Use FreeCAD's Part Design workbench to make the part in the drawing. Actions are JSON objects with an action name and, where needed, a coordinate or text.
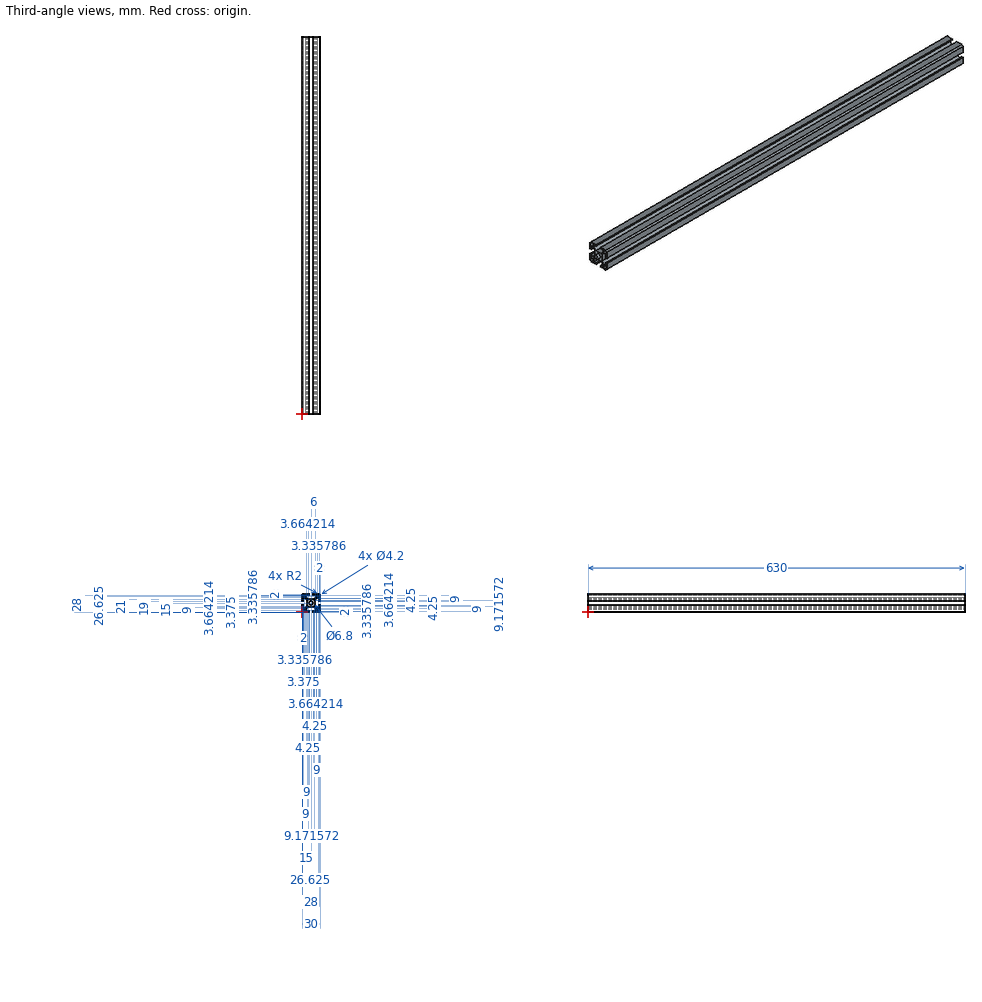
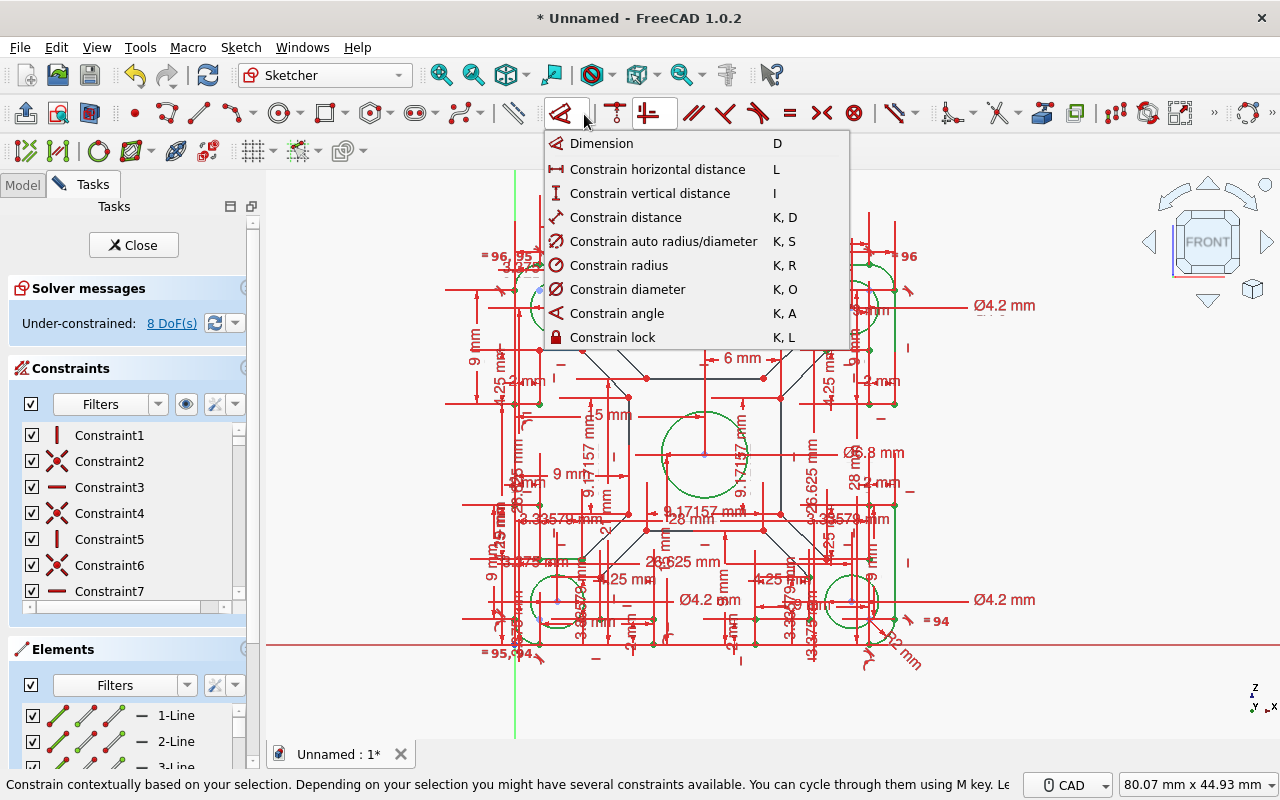
{"action": "left_click", "coordinate": [697, 169]}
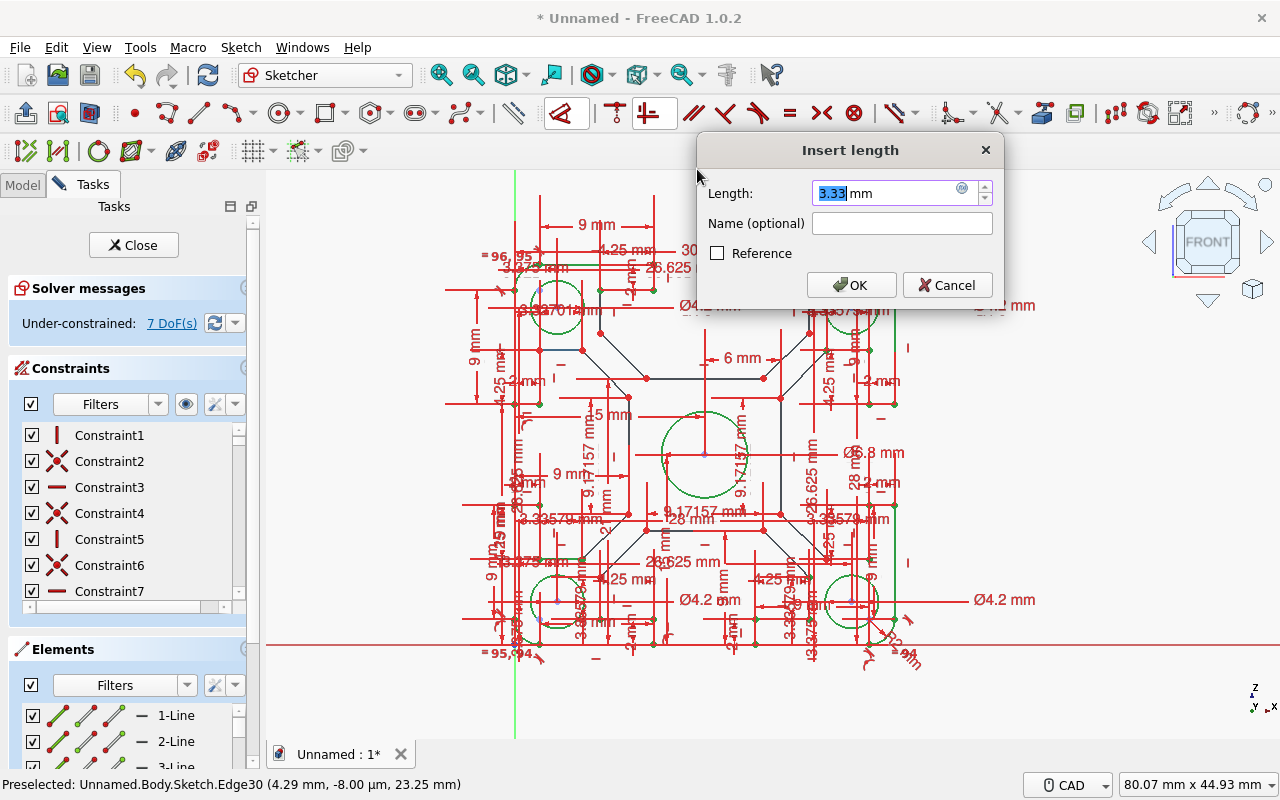
{"action": "type", "text": "3.335786"}
{"action": "key", "text": "Return"}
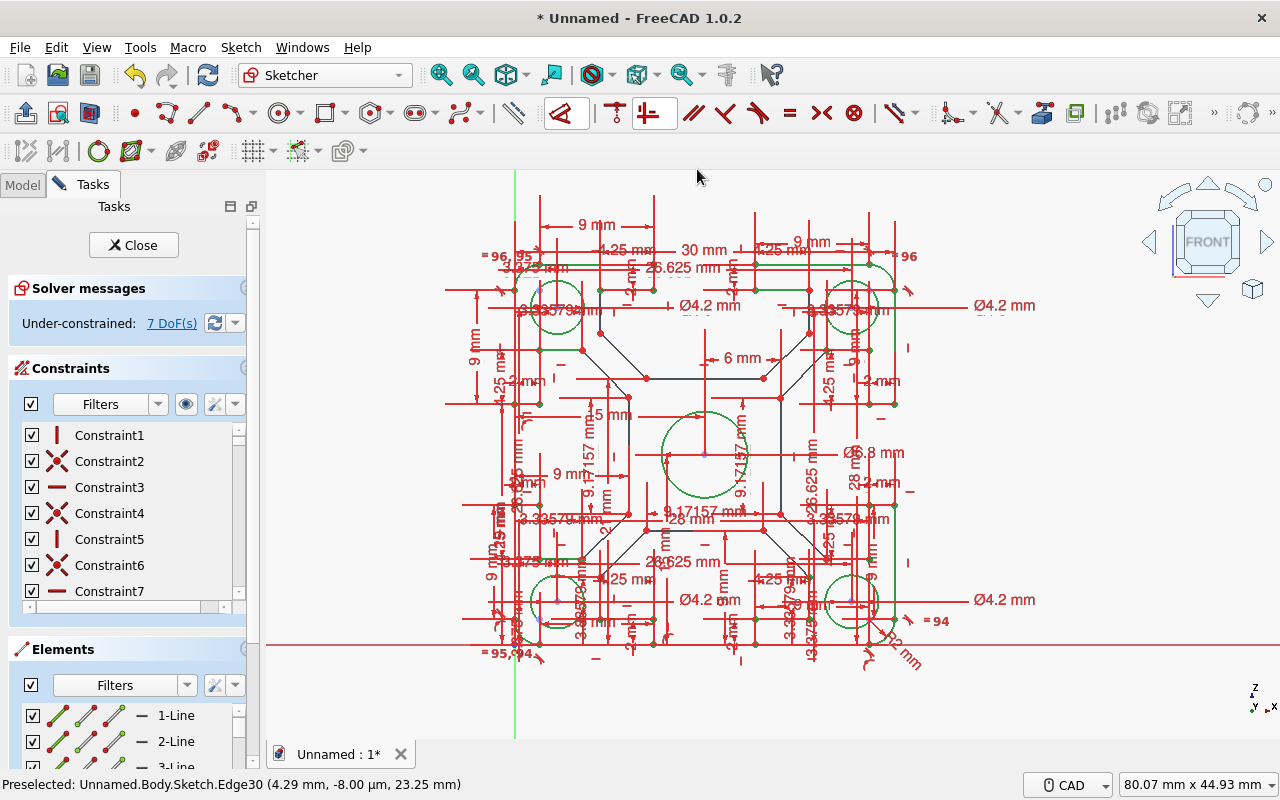
{"action": "left_click", "coordinate": [600, 303]}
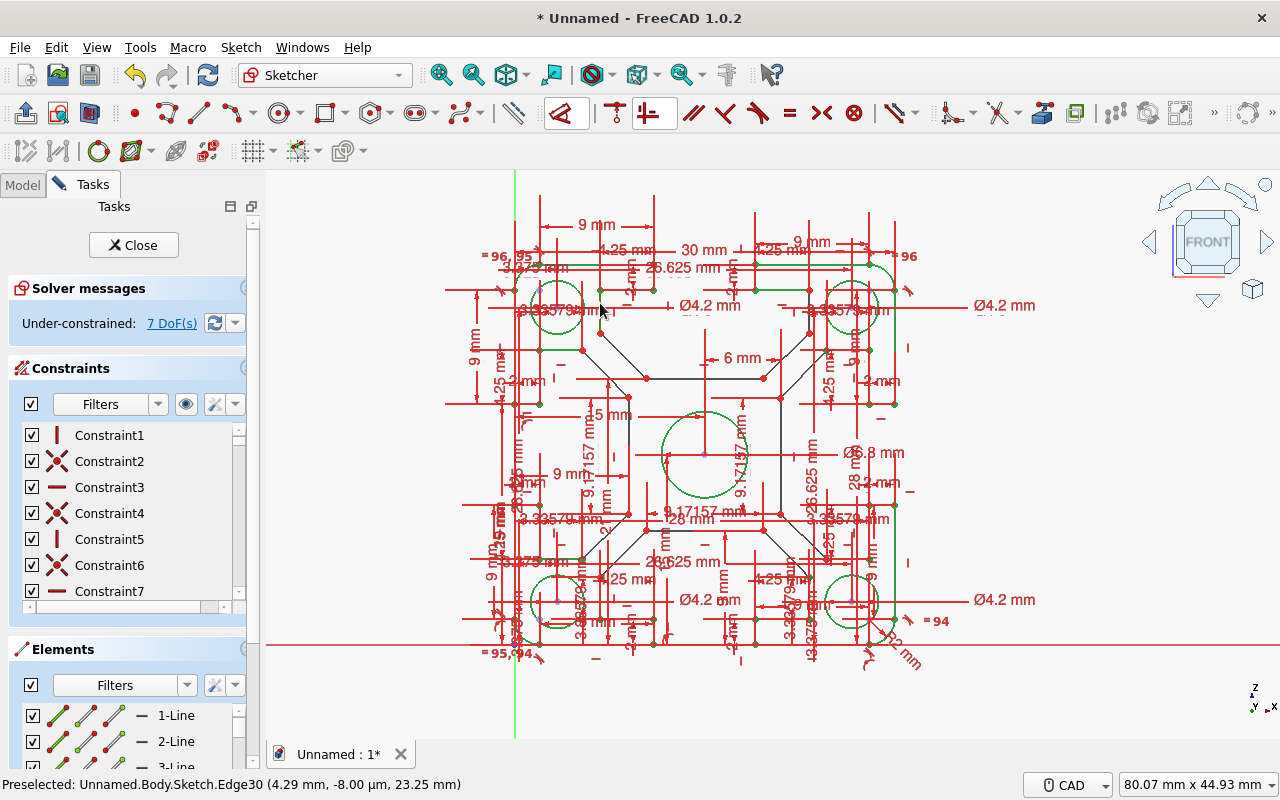
{"action": "left_click", "coordinate": [584, 114]}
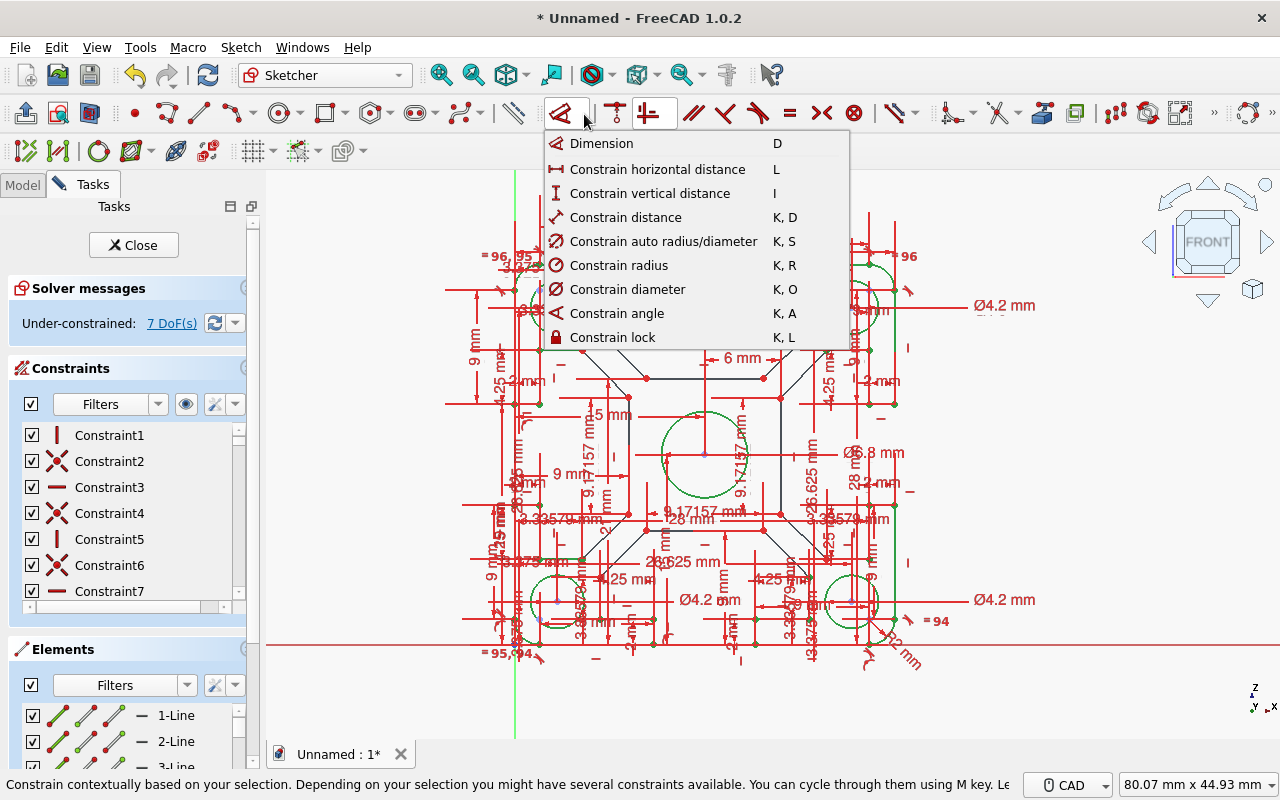
{"action": "left_click", "coordinate": [697, 193]}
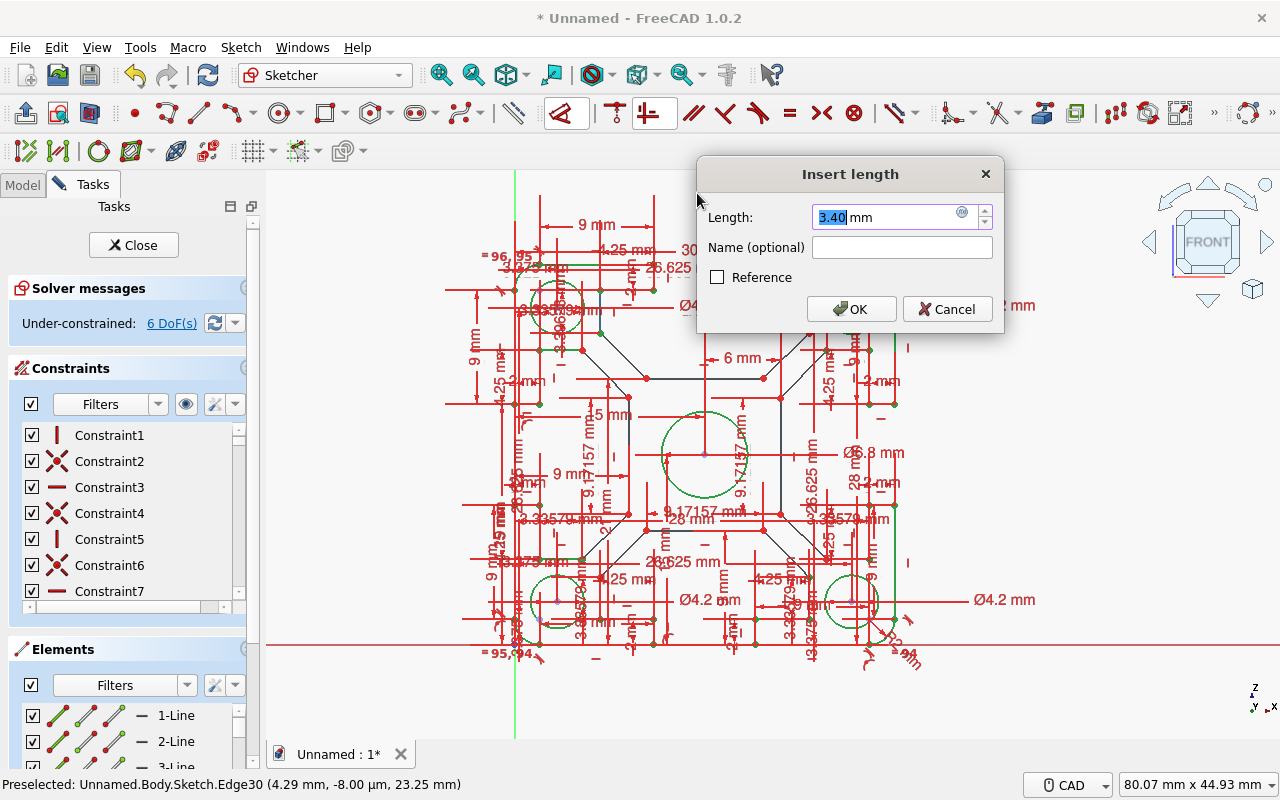
{"action": "type", "text": "3.335786"}
{"action": "key", "text": "Return"}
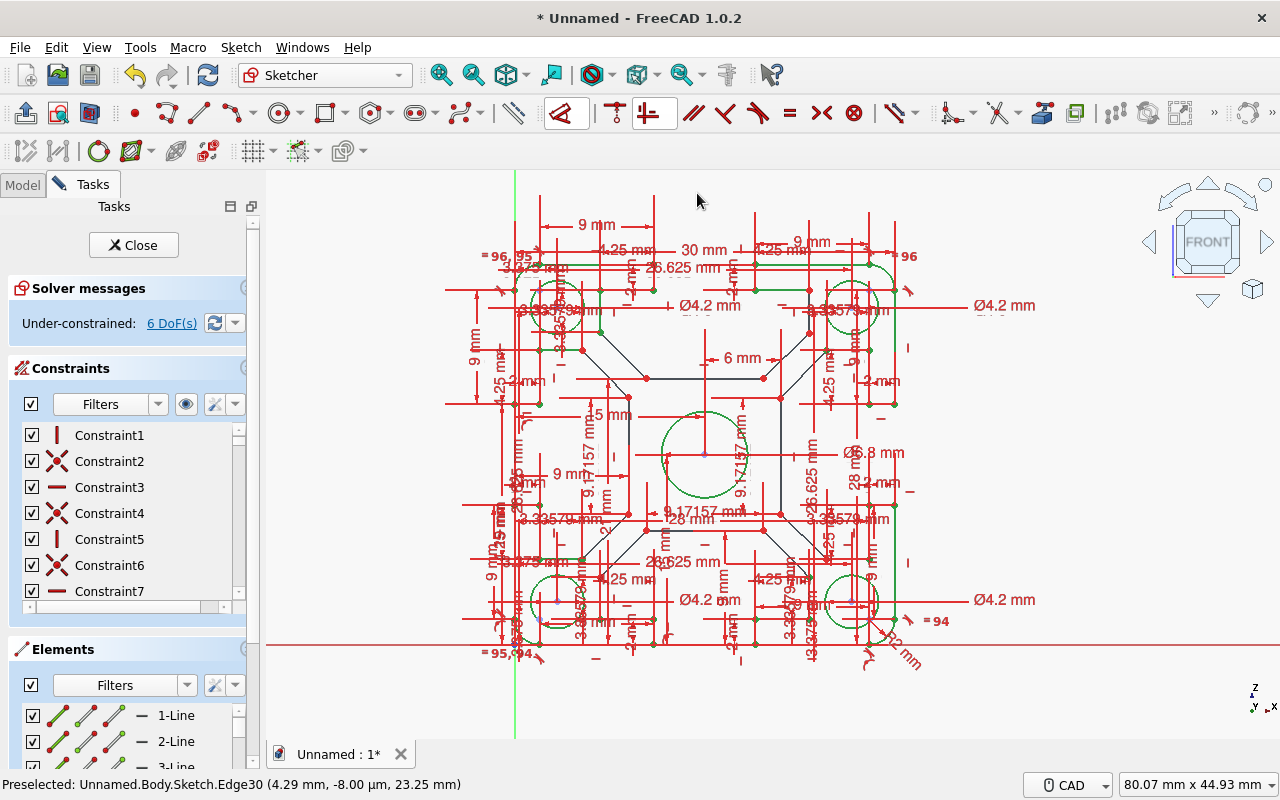
{"action": "left_click", "coordinate": [681, 379]}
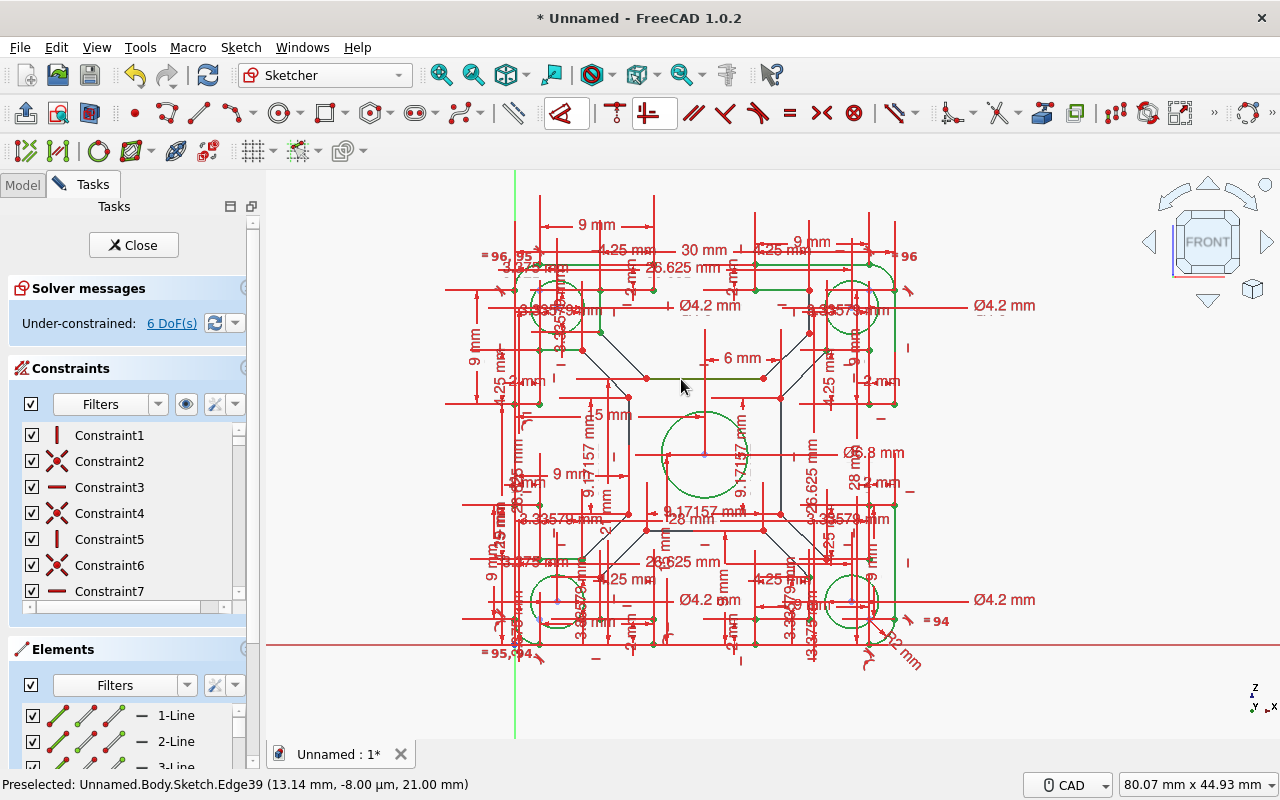
{"action": "key", "text": "l"}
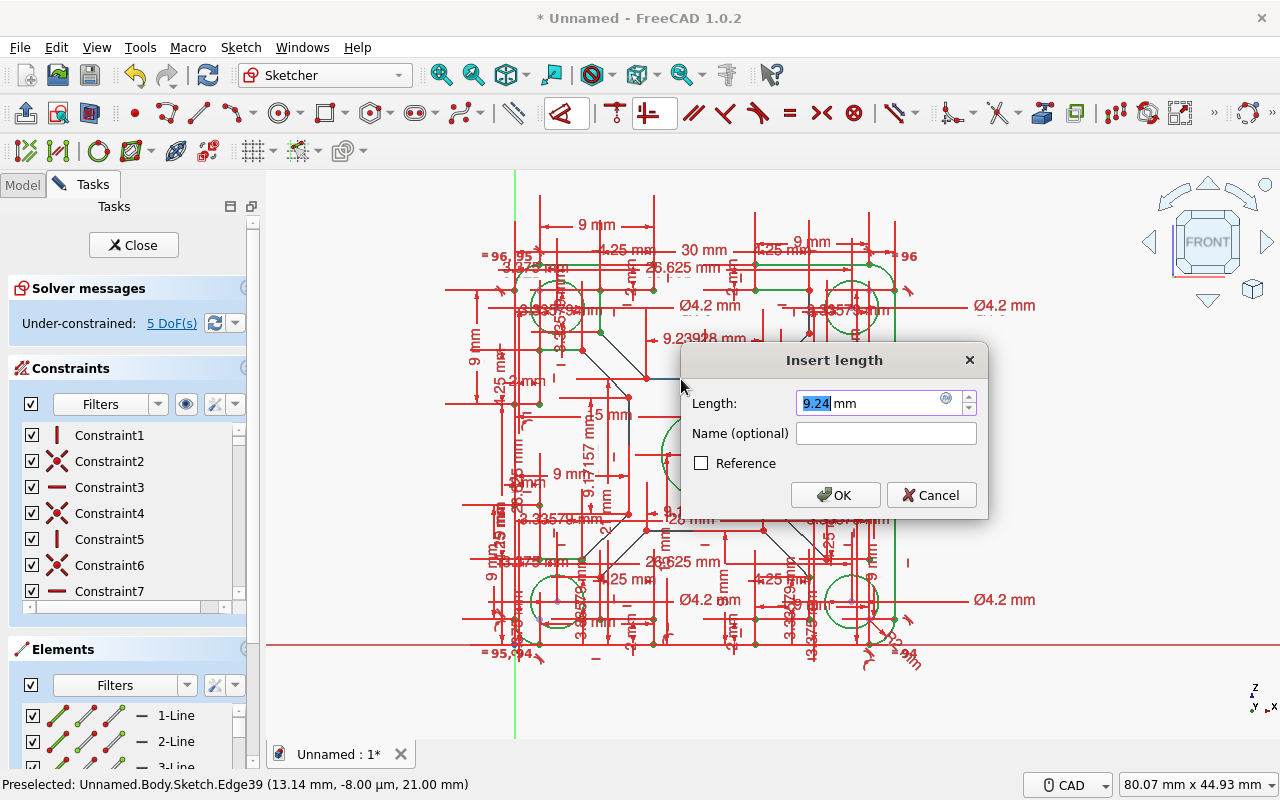
{"action": "type", "text": "9.171572"}
{"action": "key", "text": "Return"}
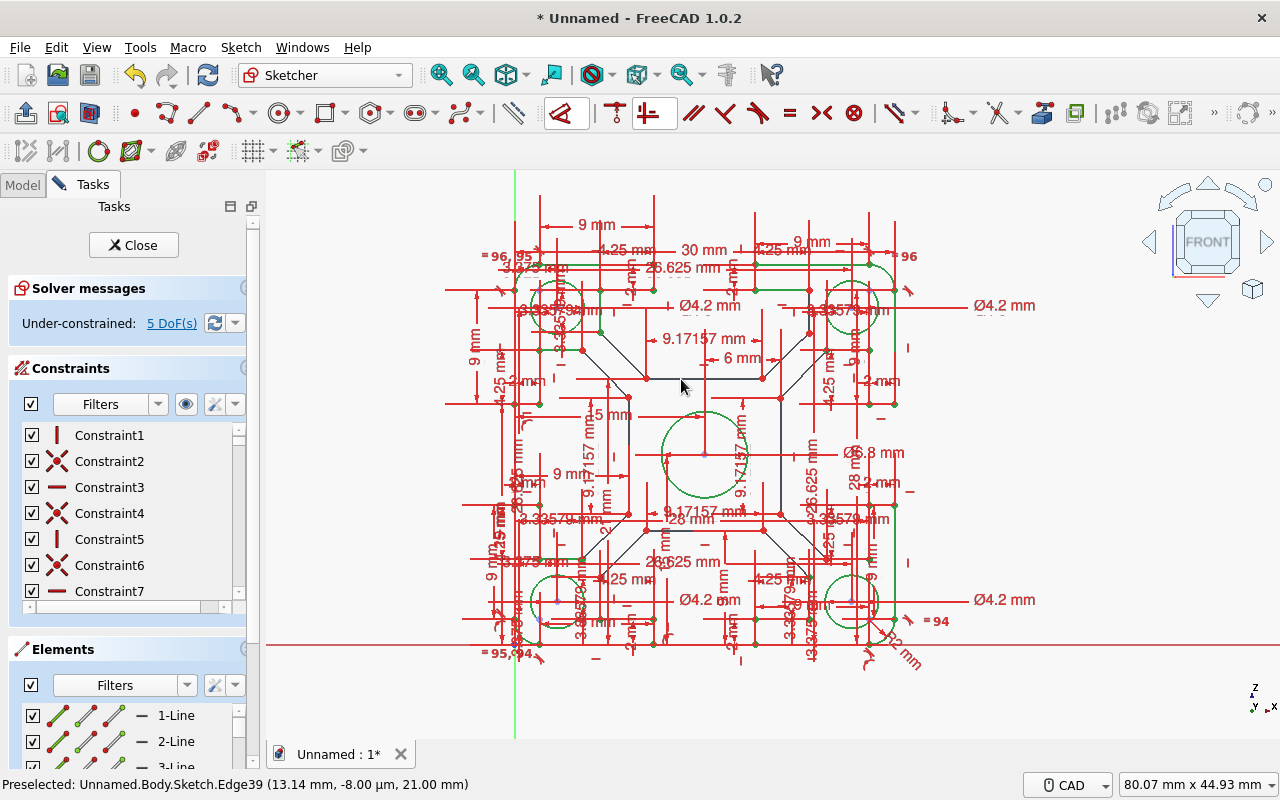
{"action": "left_click", "coordinate": [809, 320]}